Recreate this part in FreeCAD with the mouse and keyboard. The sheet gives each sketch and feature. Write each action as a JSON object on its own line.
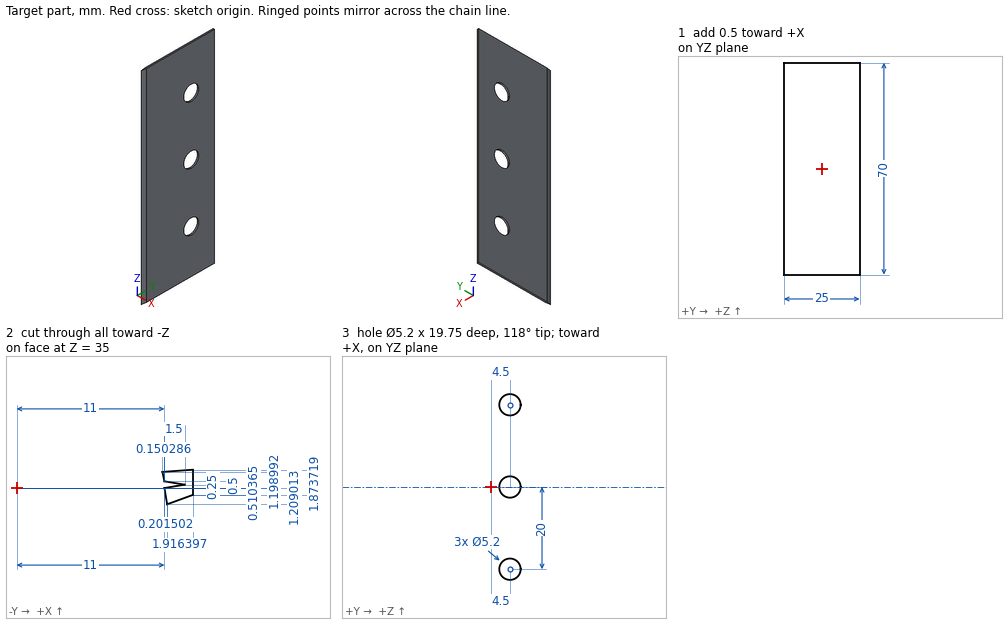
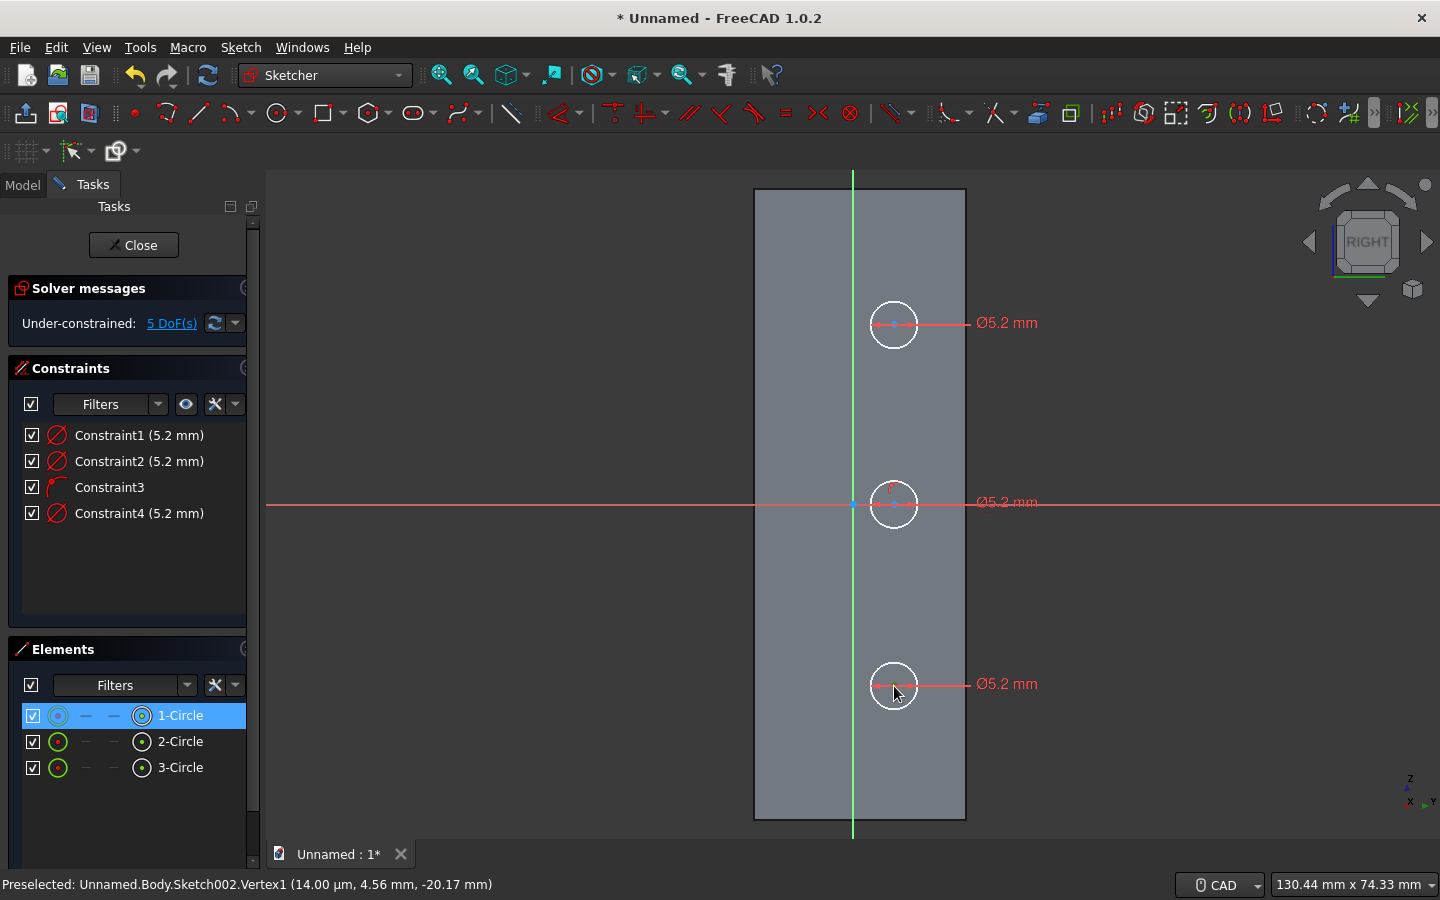
{"action": "left_click", "coordinate": [894, 325]}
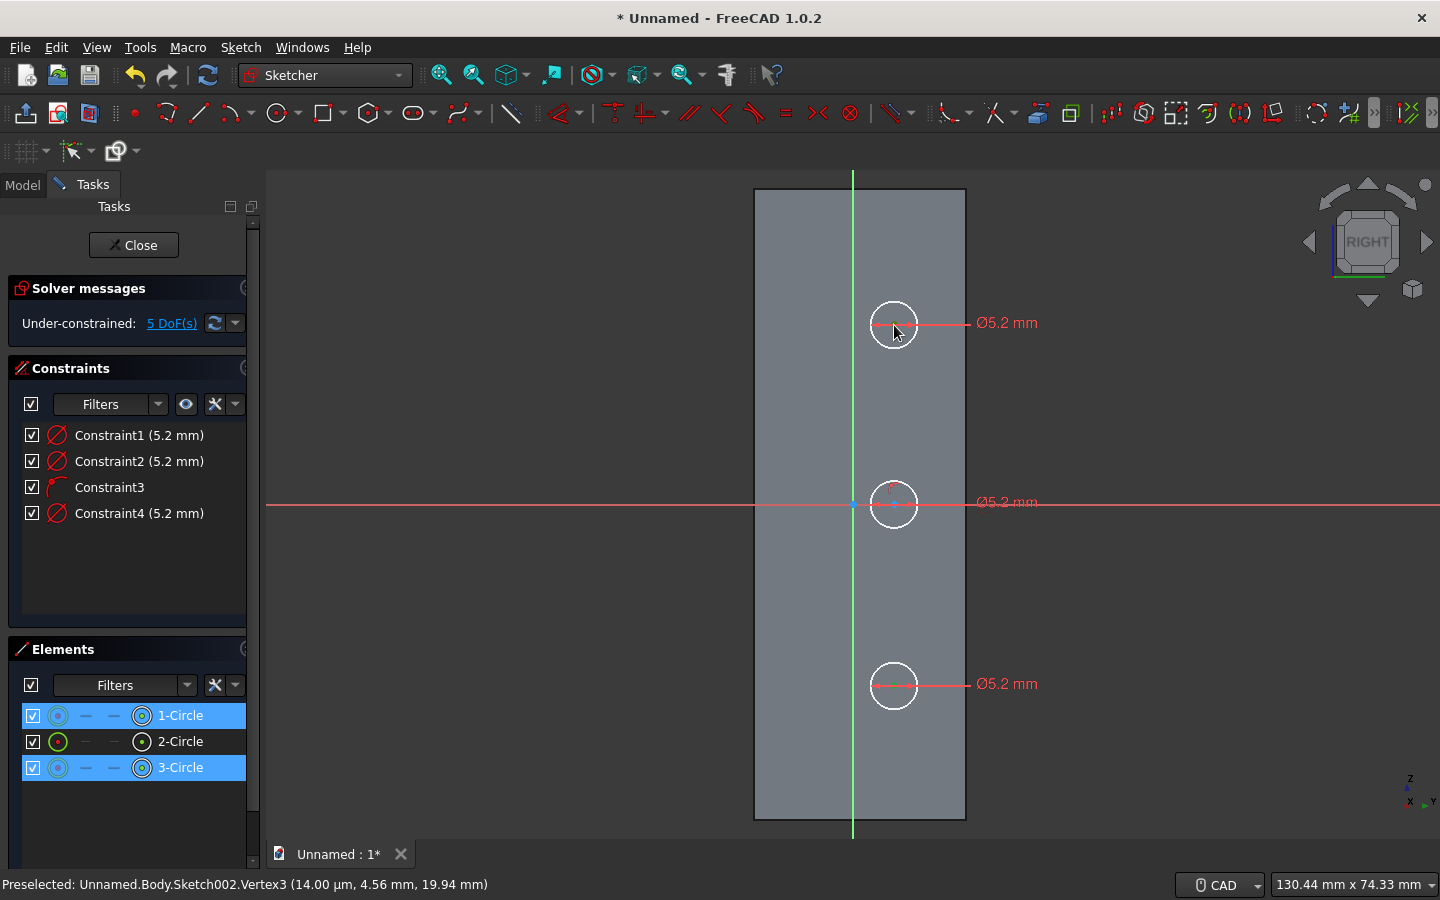
{"action": "left_click", "coordinate": [364, 504]}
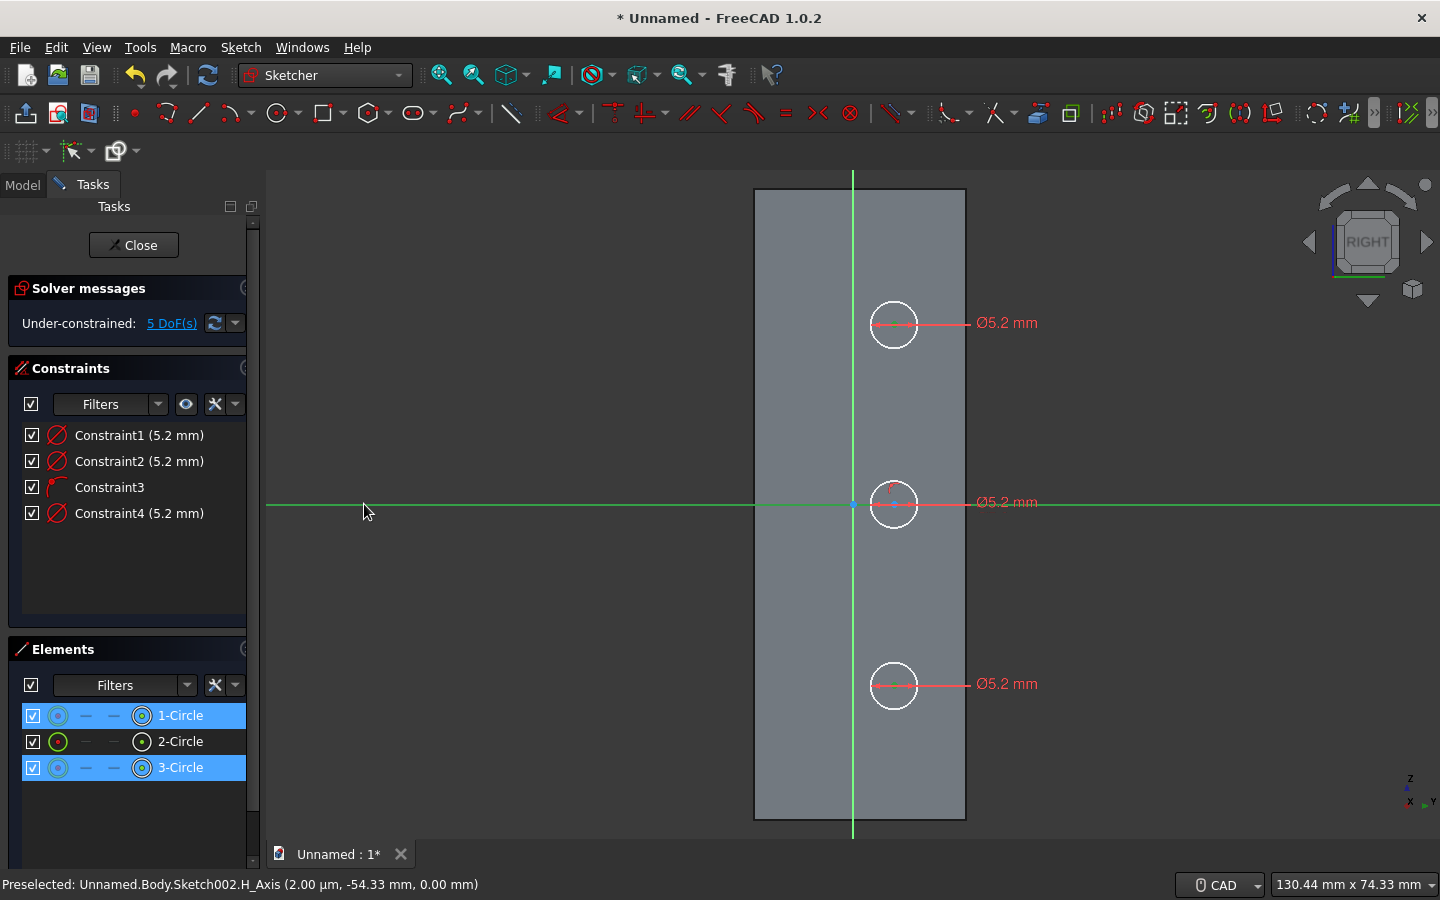
{"action": "key", "text": "s"}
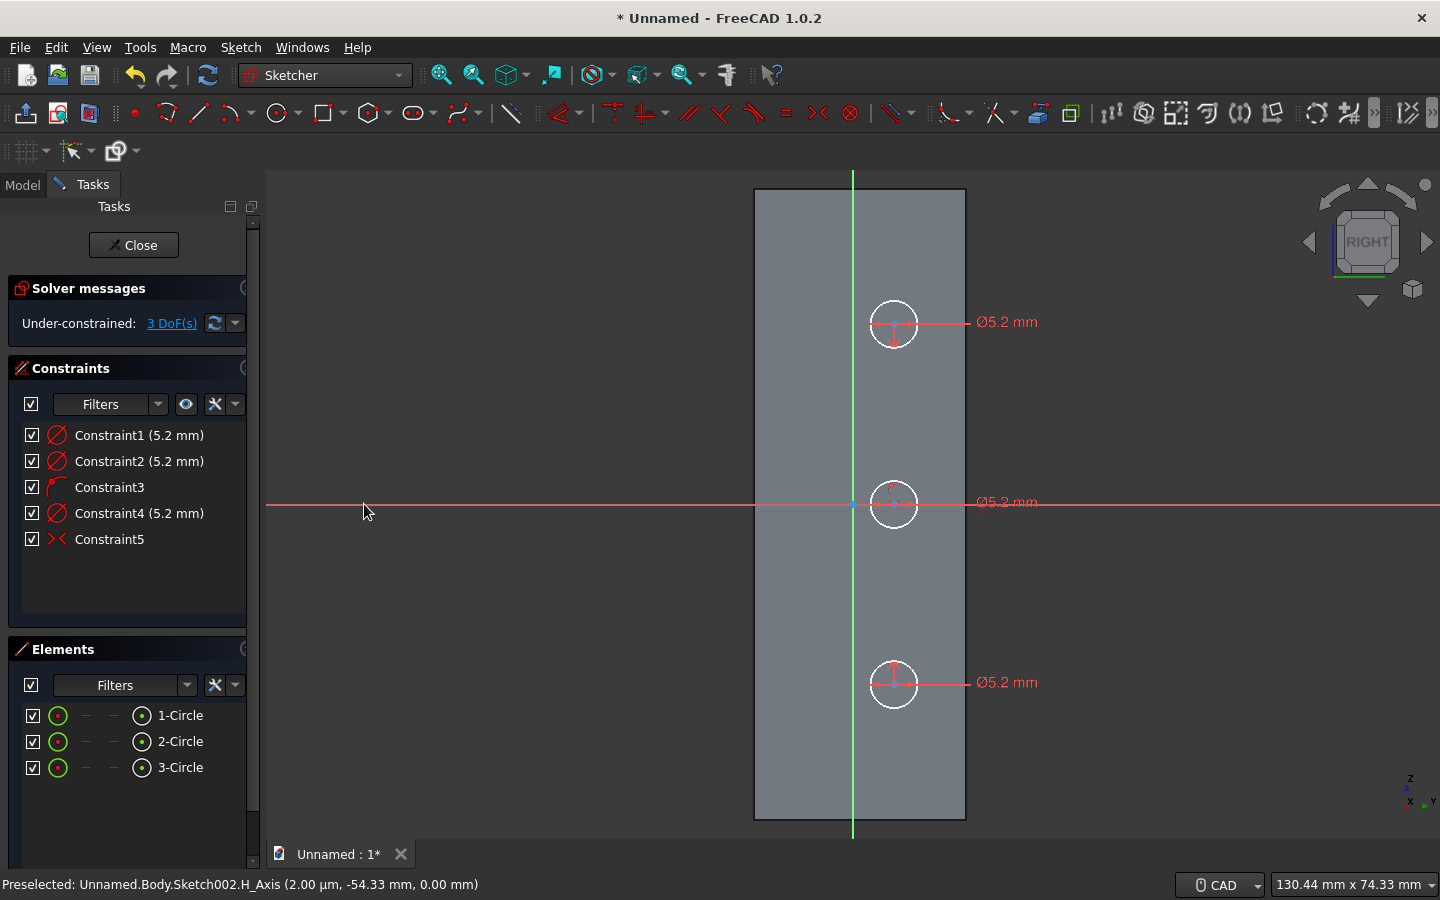
{"action": "left_click", "coordinate": [558, 114]}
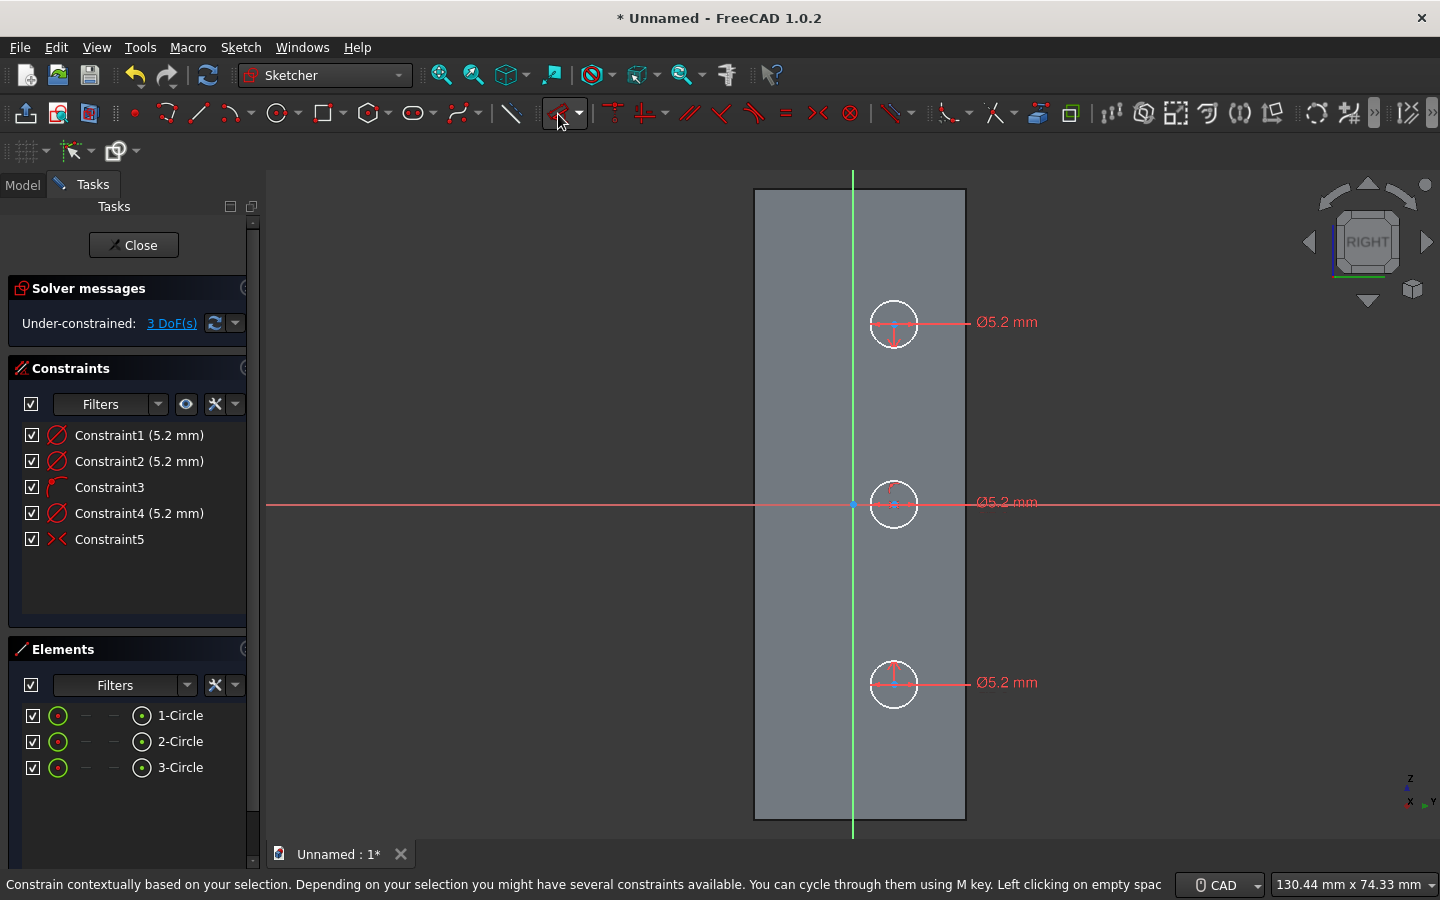
{"action": "left_click", "coordinate": [894, 685]}
{"action": "left_click", "coordinate": [819, 595]}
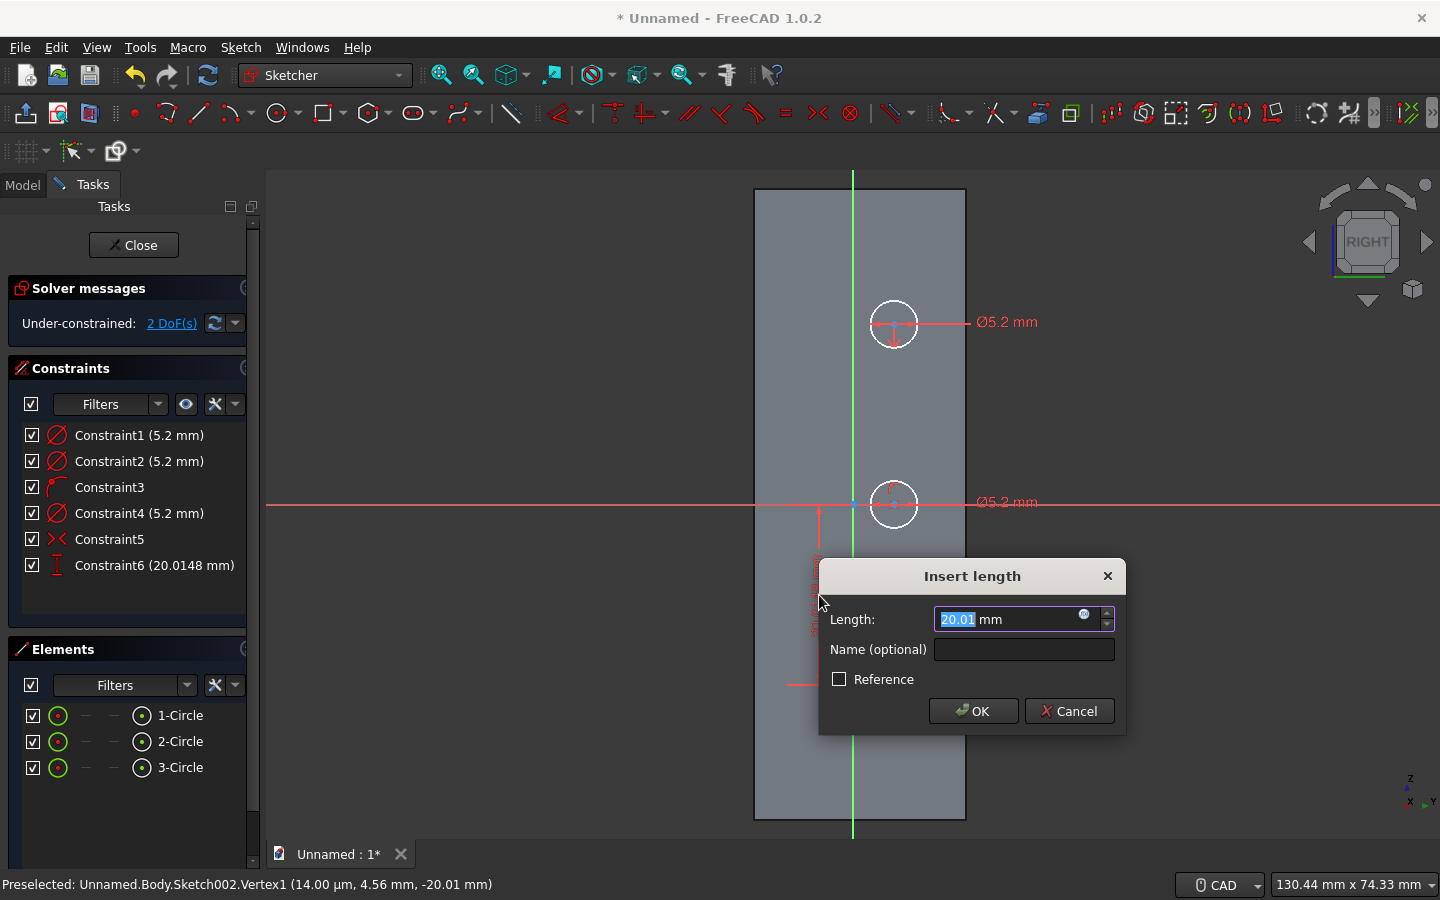
{"action": "type", "text": "20"}
{"action": "key", "text": "Return"}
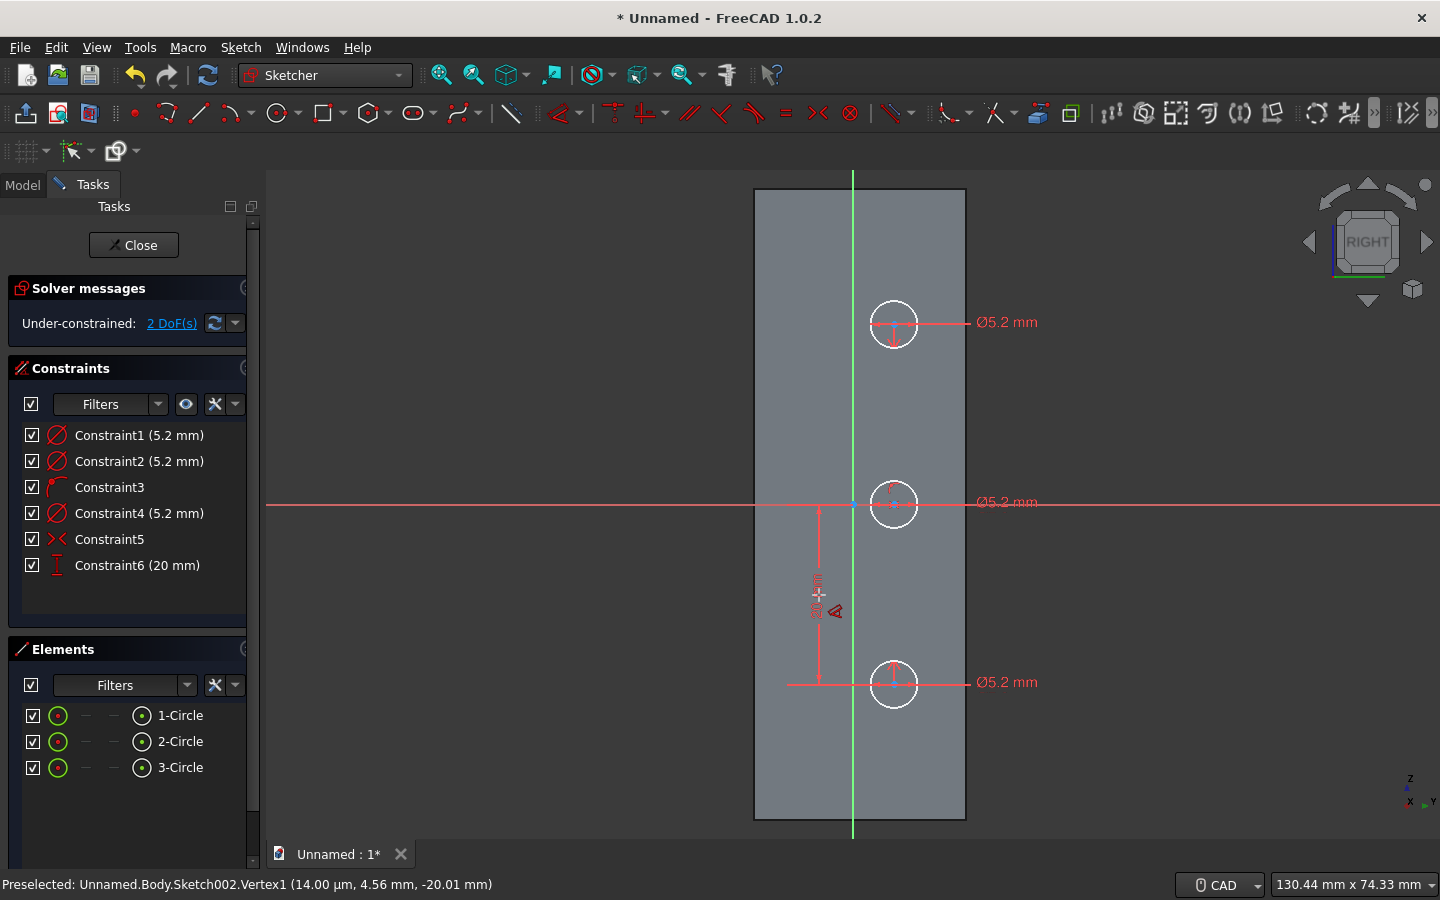
{"action": "left_click", "coordinate": [894, 685]}
{"action": "left_click", "coordinate": [873, 719]}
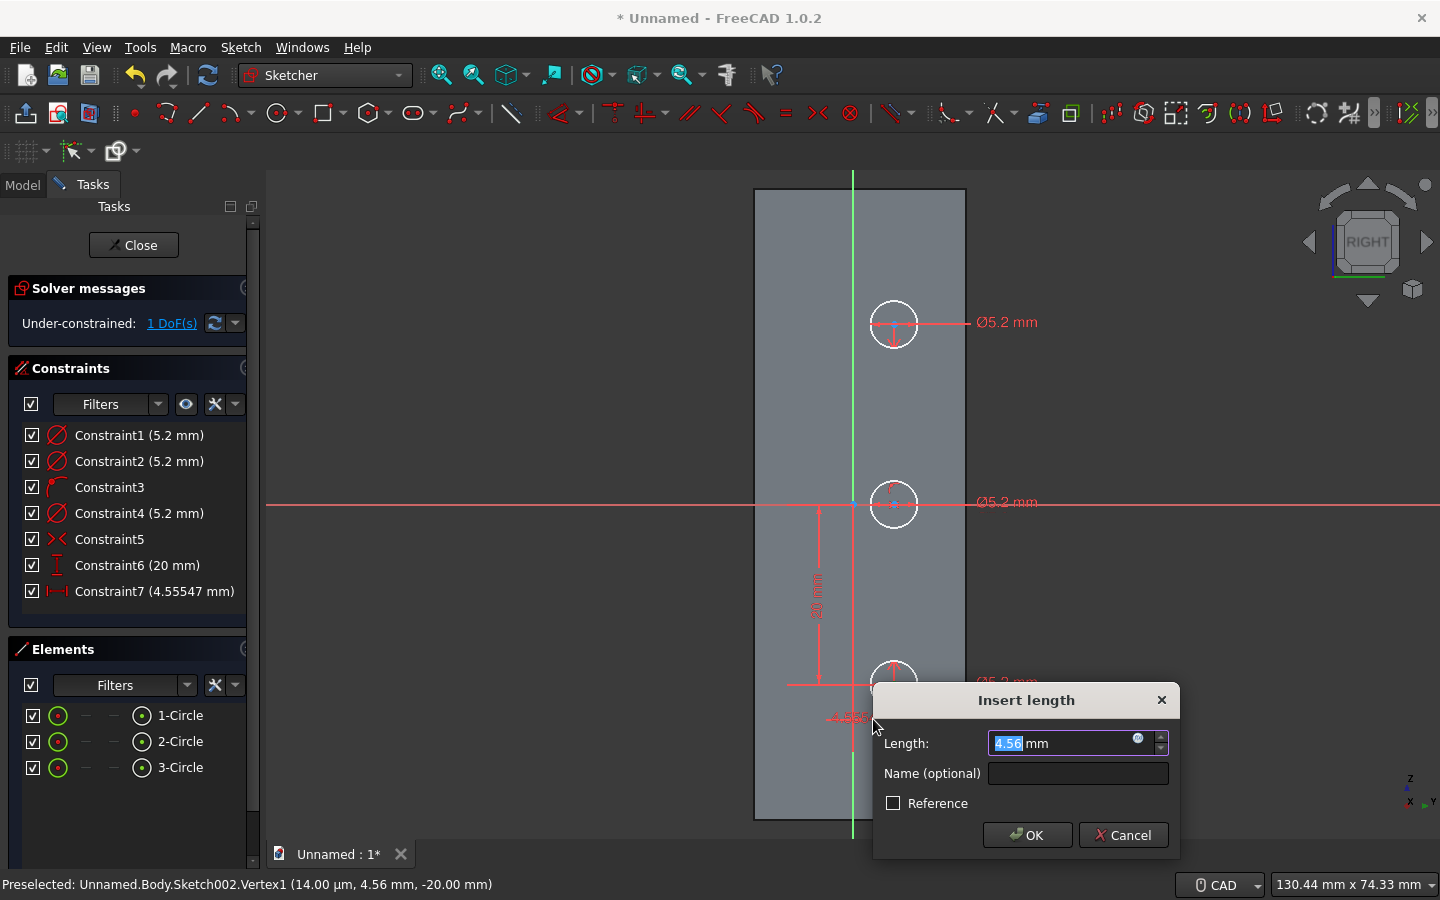
{"action": "type", "text": "4.5"}
{"action": "key", "text": "Return"}